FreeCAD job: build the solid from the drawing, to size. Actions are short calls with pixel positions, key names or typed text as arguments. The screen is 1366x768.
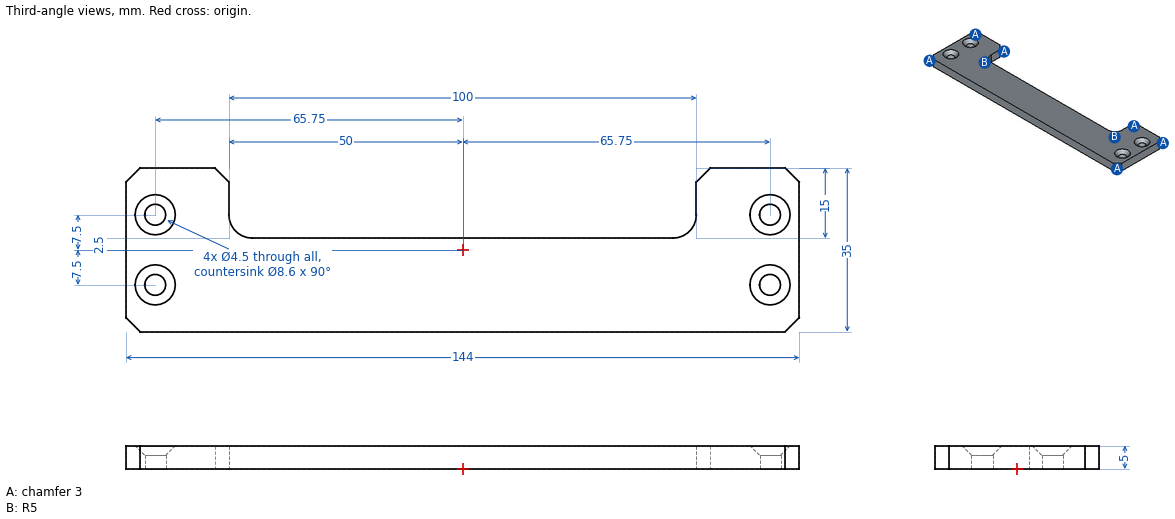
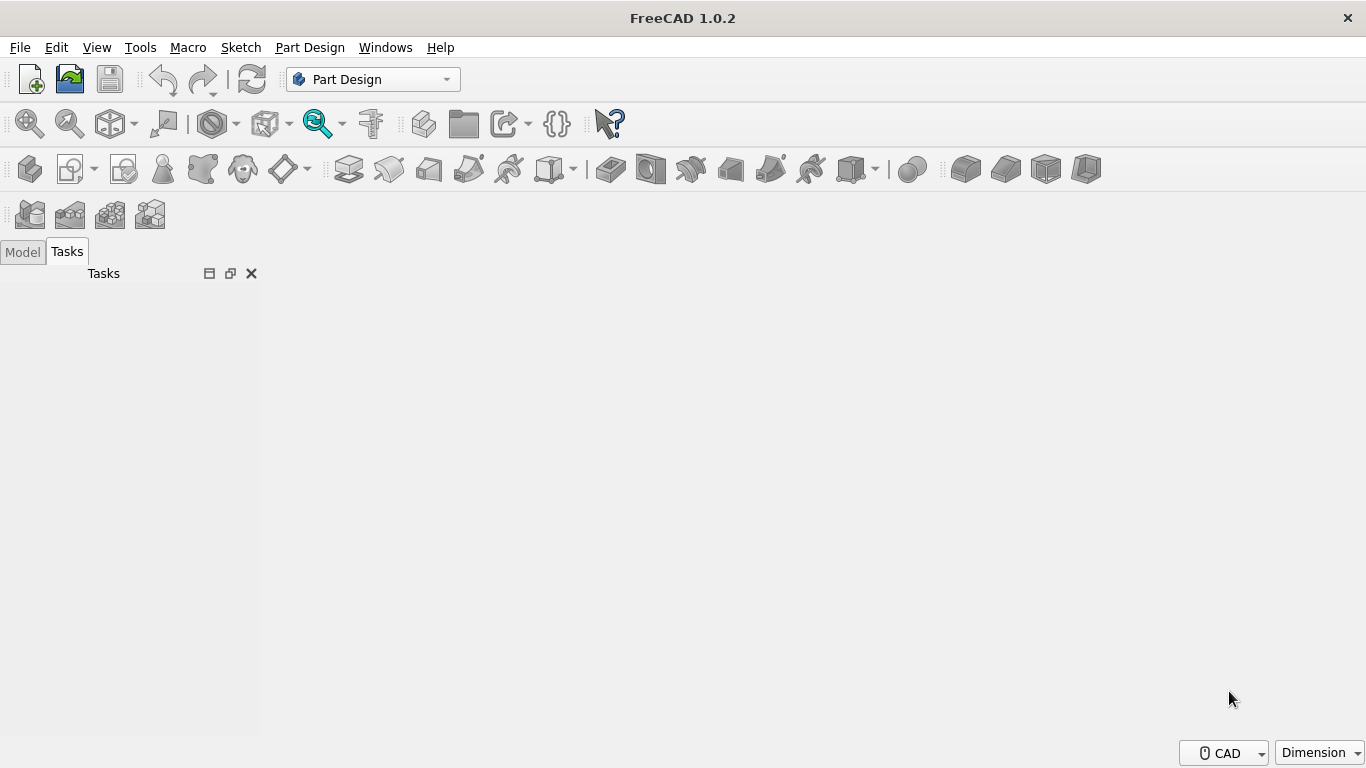
key(ctrl+n)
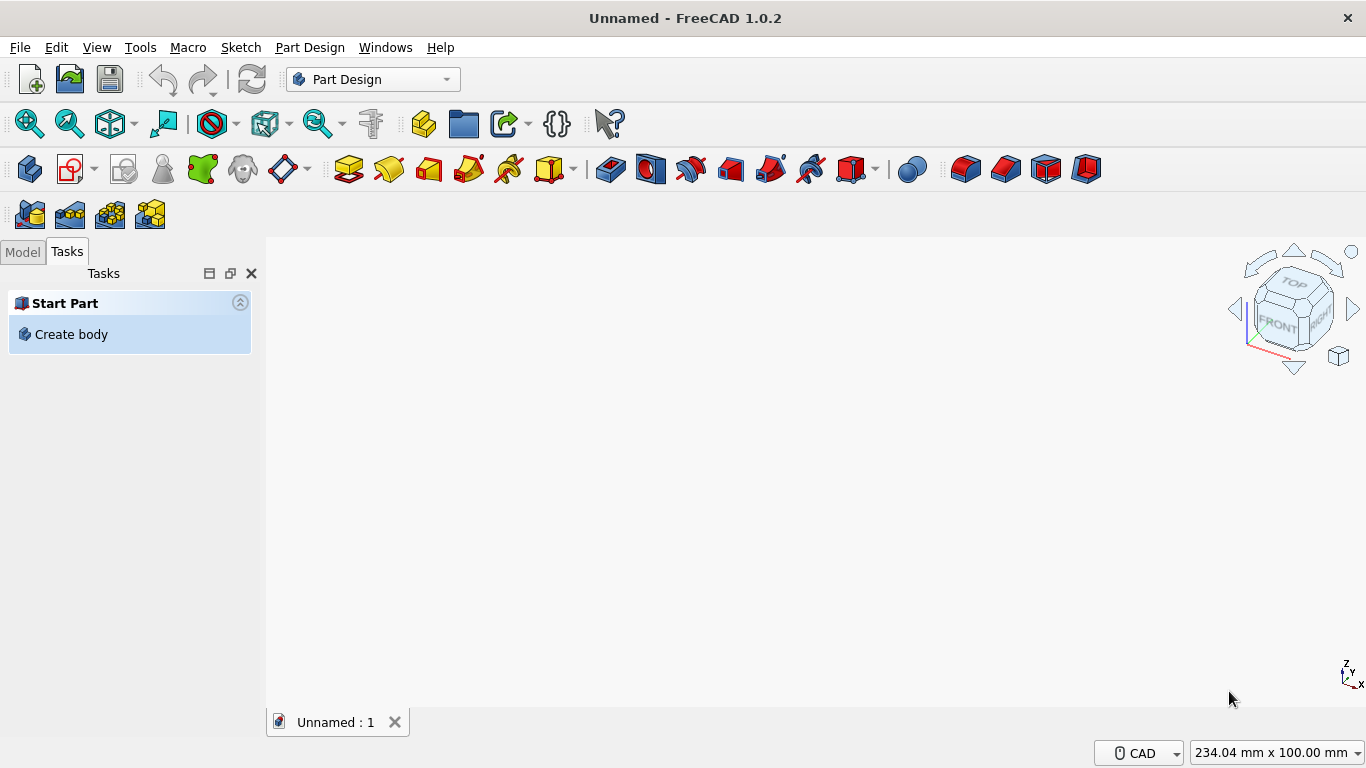
click(70, 170)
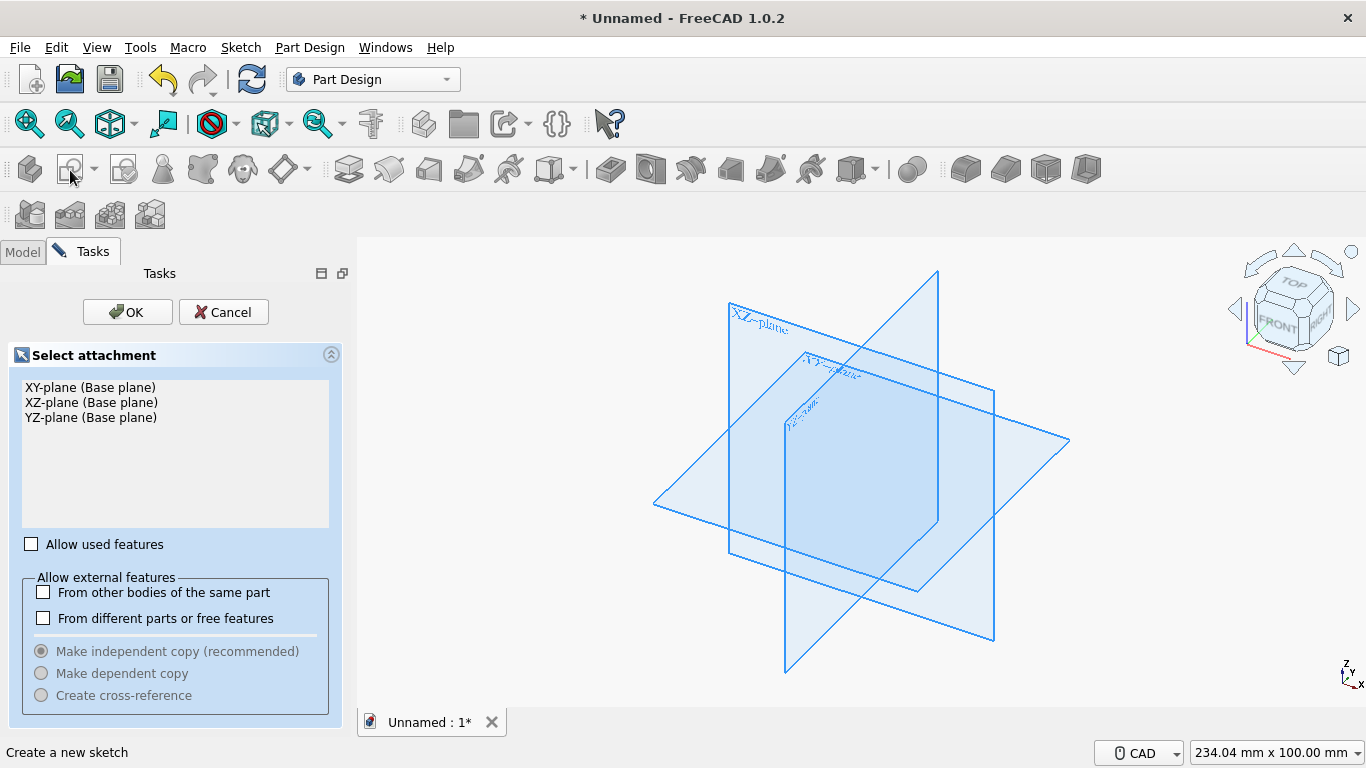
click(82, 388)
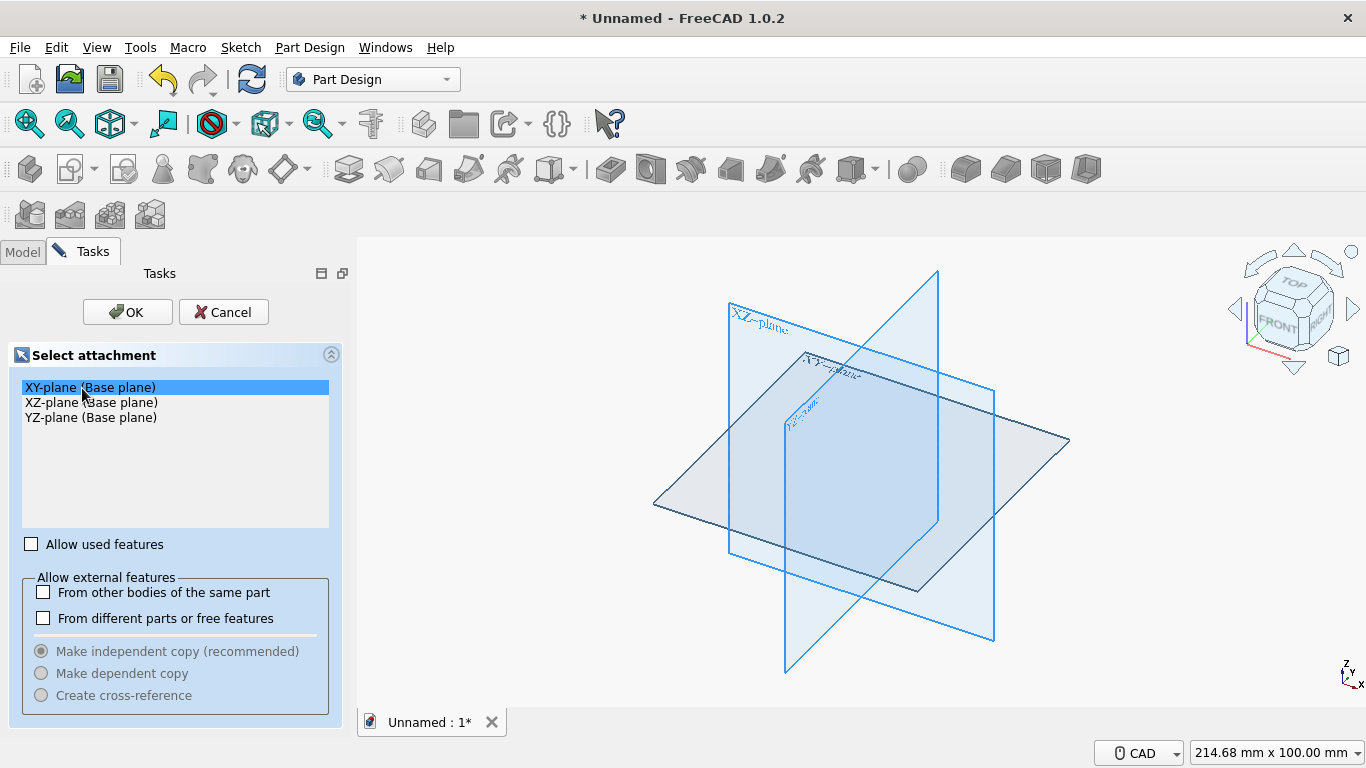
click(128, 312)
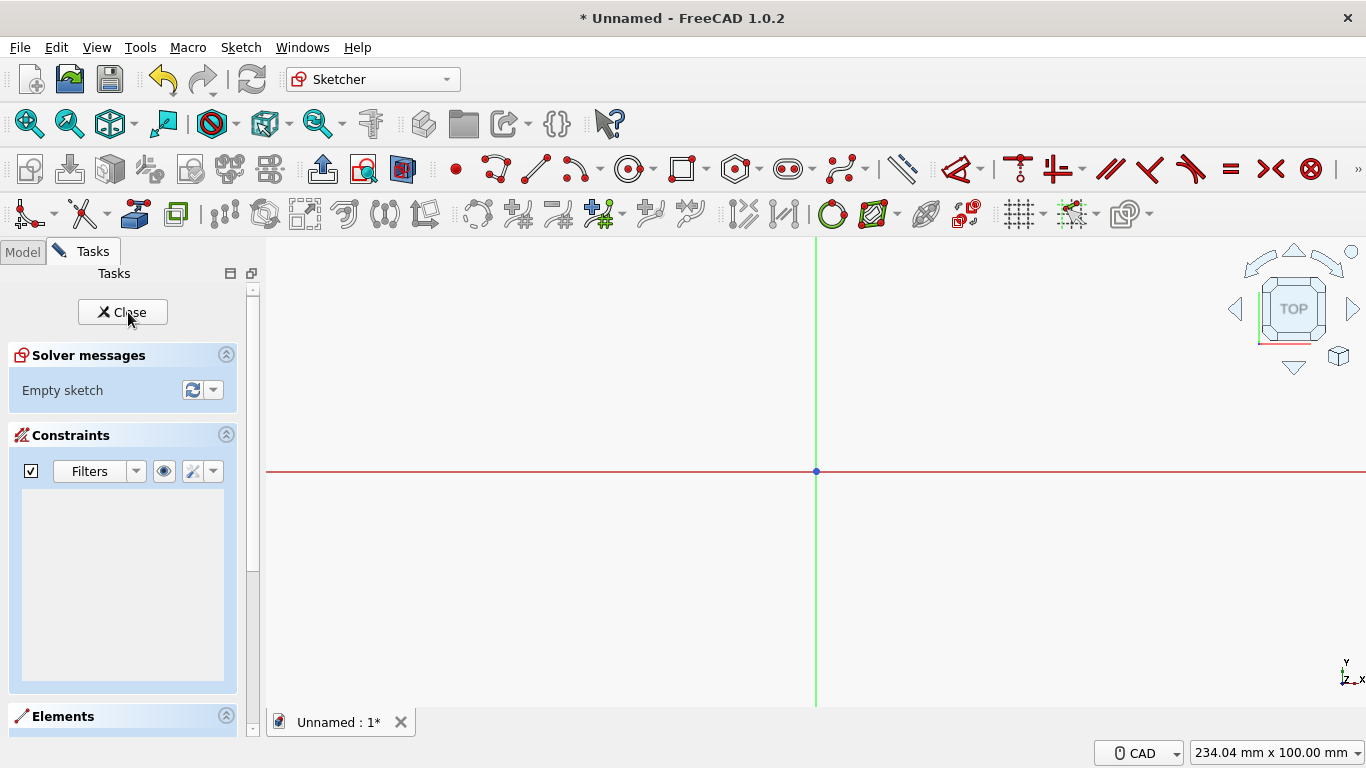
key(g)
key(v)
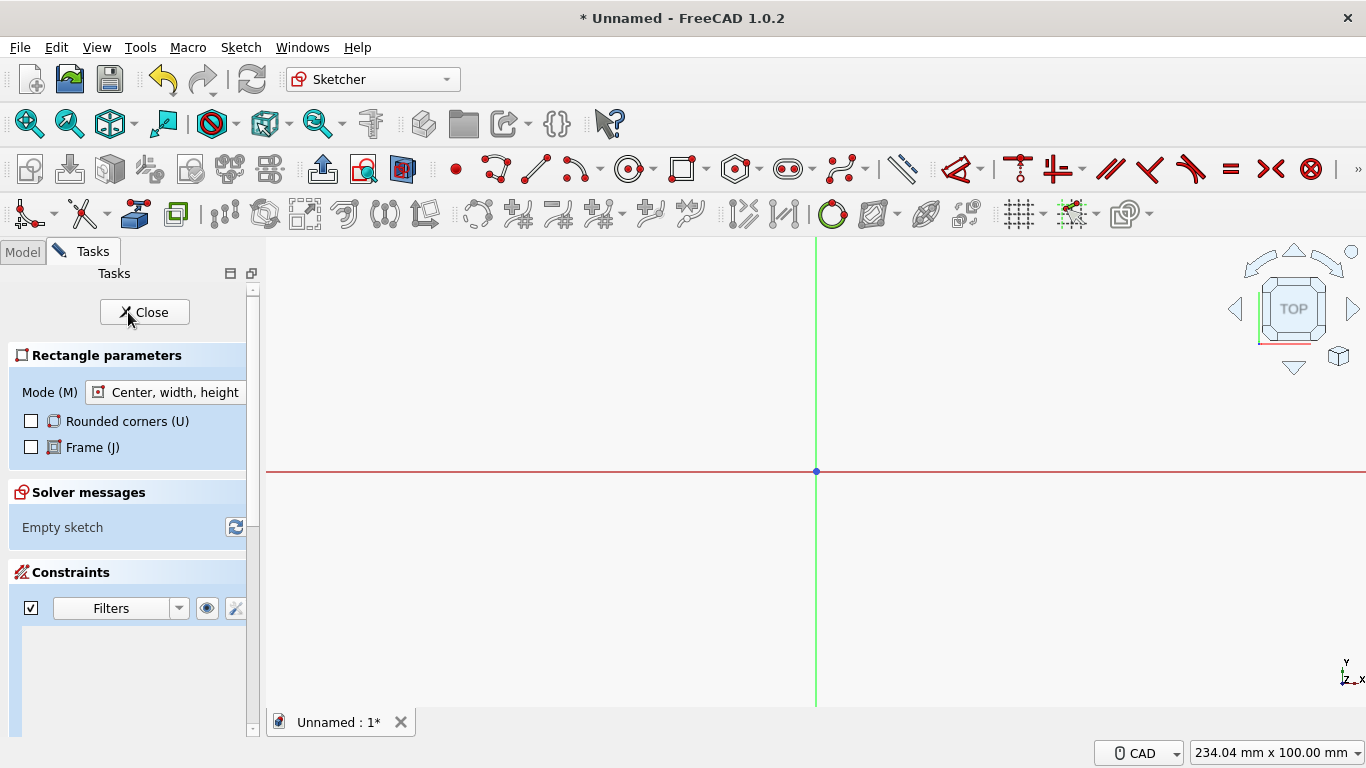
click(816, 472)
move(1154, 390)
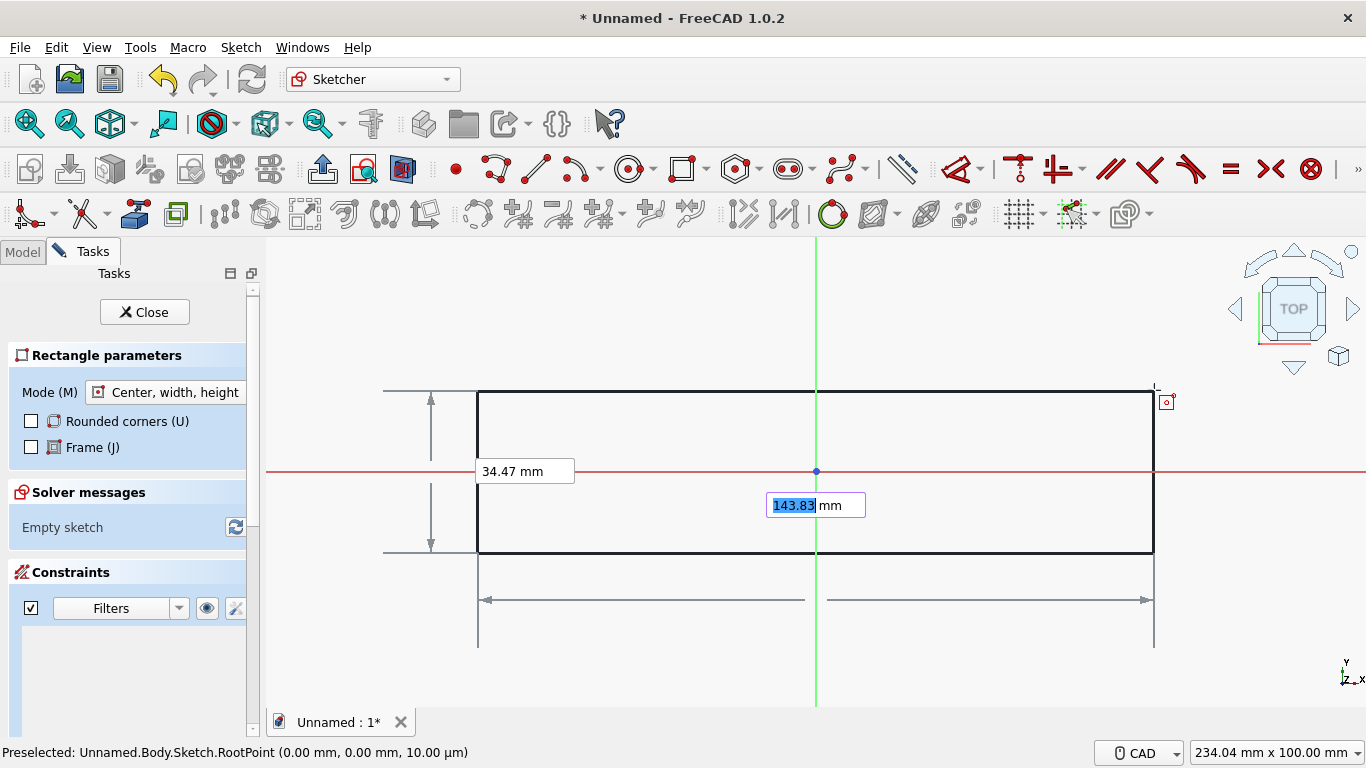
text(144)
key(Tab)
text(35)
key(Return)
key(Escape)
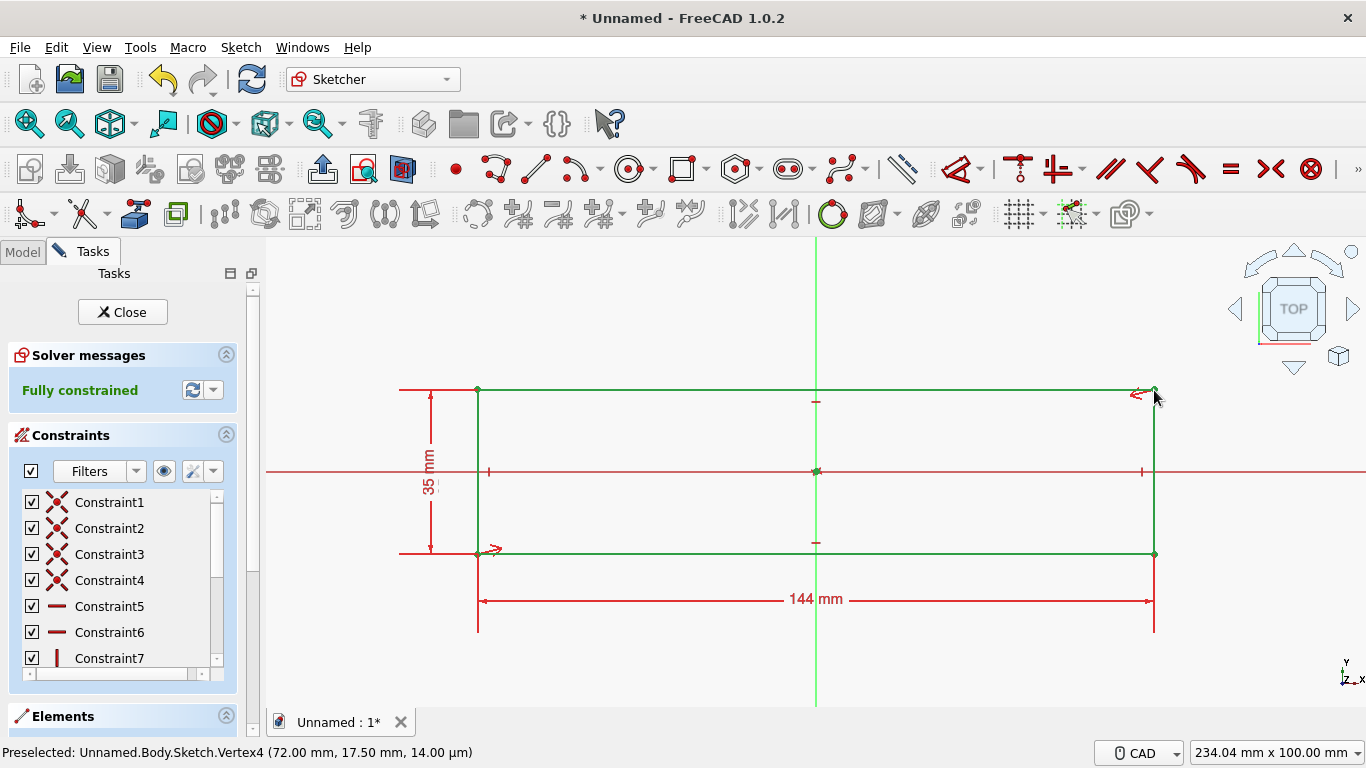
click(123, 312)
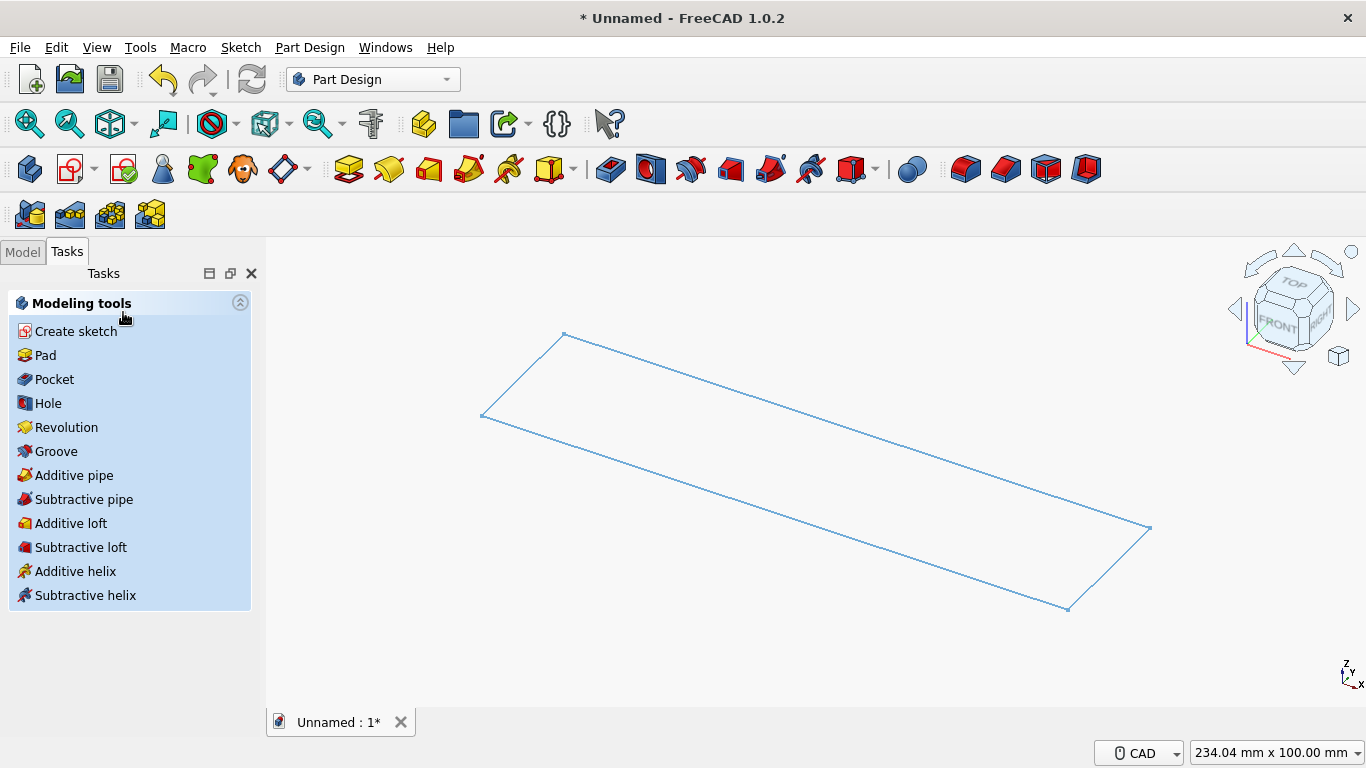
click(350, 170)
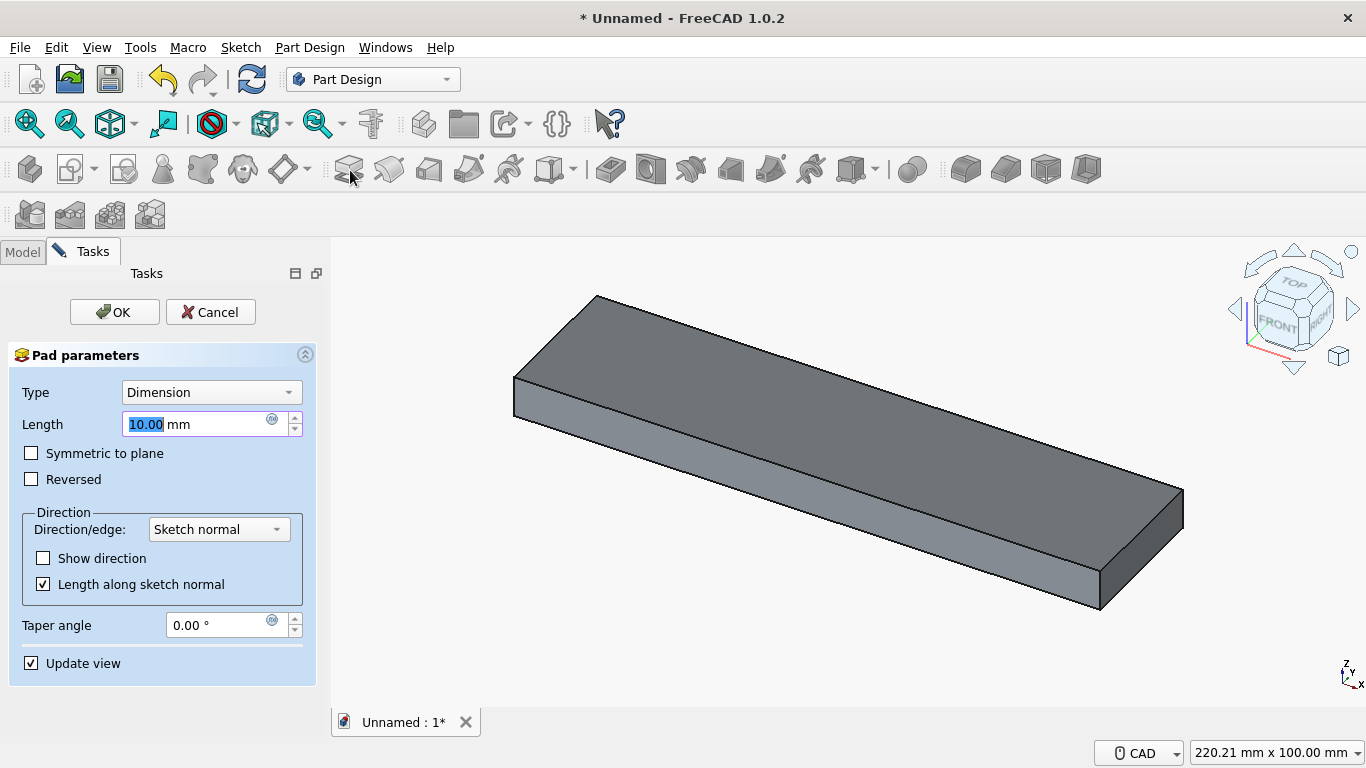
text(5)
key(Tab)